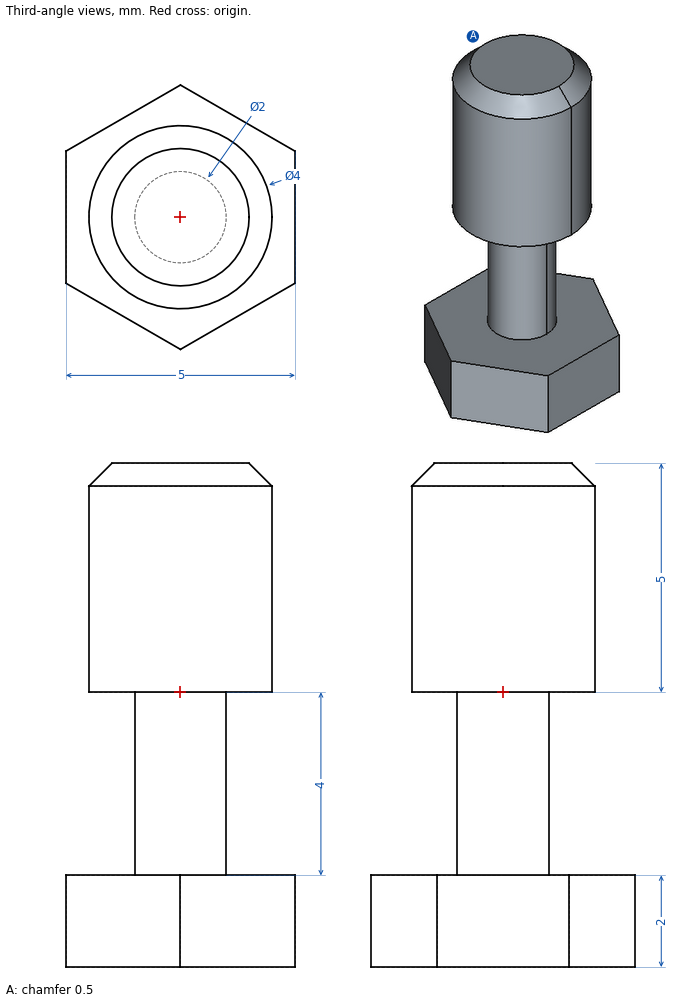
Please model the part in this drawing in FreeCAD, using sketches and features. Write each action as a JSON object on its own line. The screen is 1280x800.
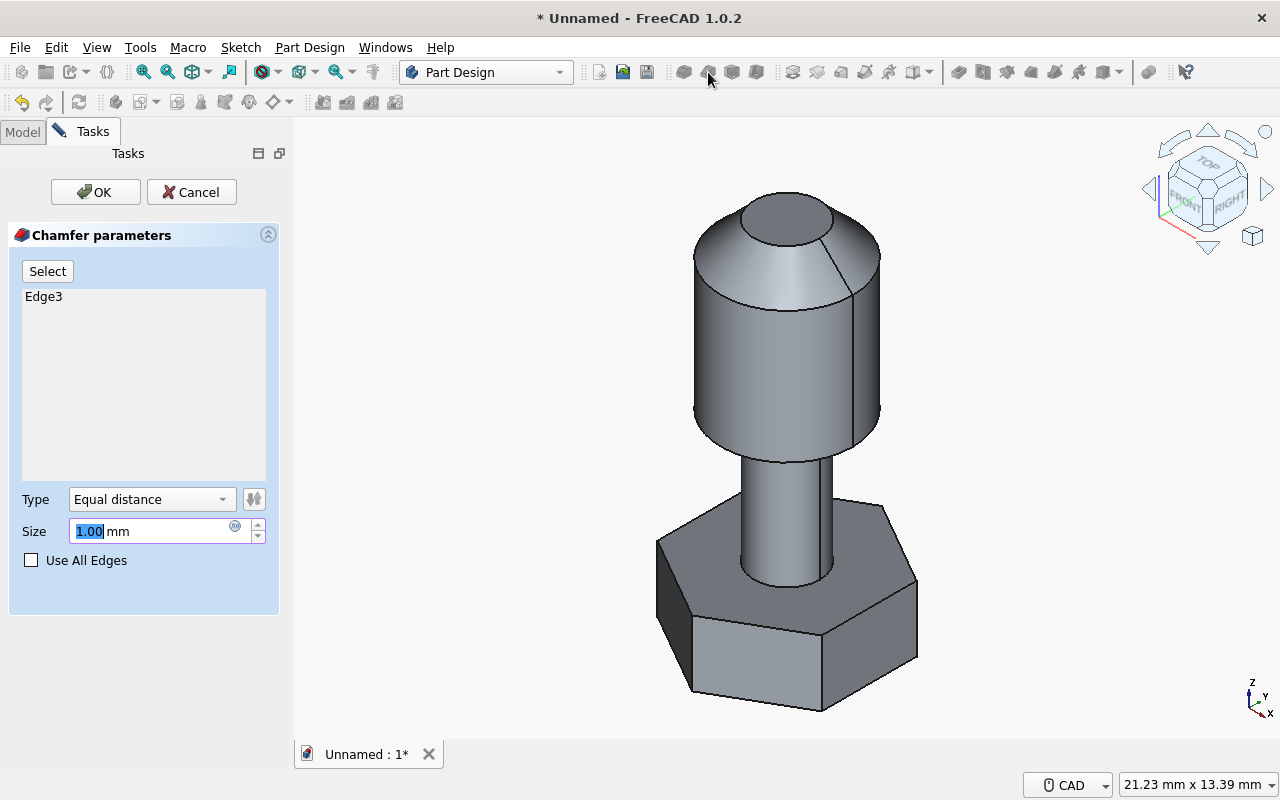
{"action": "type", "text": "0.5"}
{"action": "key", "text": "Tab"}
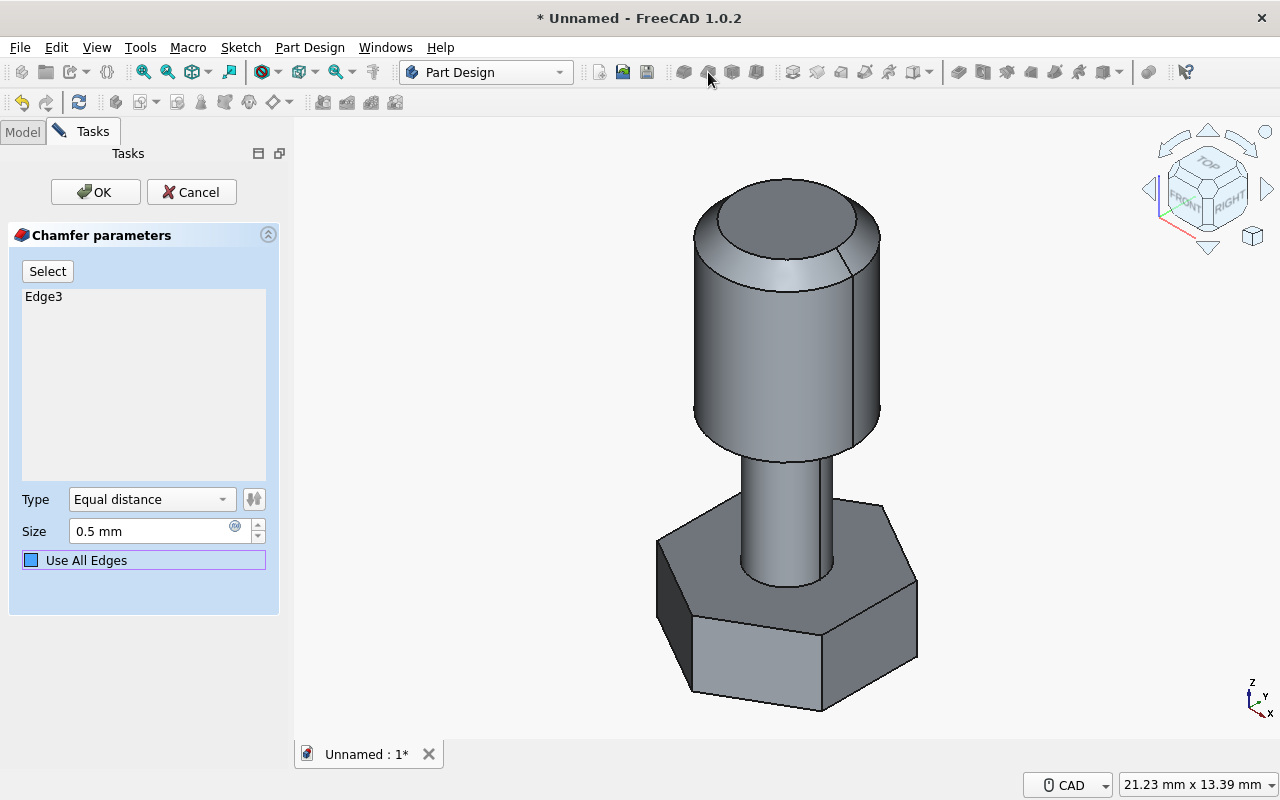
{"action": "left_click", "coordinate": [96, 192]}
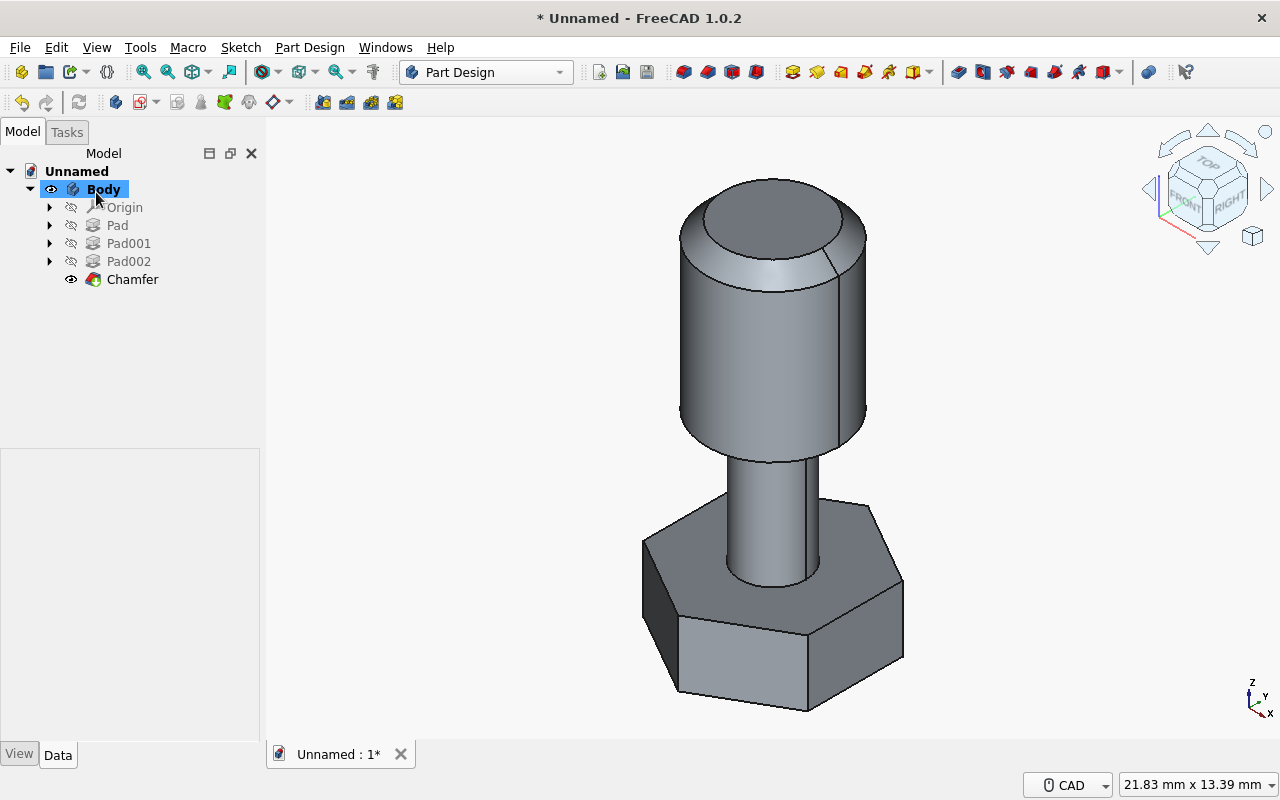
{"action": "left_click", "coordinate": [144, 72]}